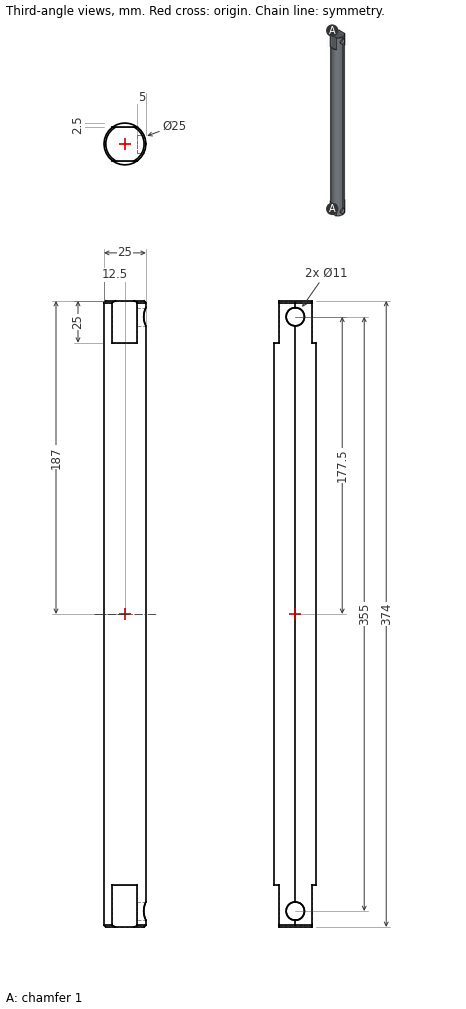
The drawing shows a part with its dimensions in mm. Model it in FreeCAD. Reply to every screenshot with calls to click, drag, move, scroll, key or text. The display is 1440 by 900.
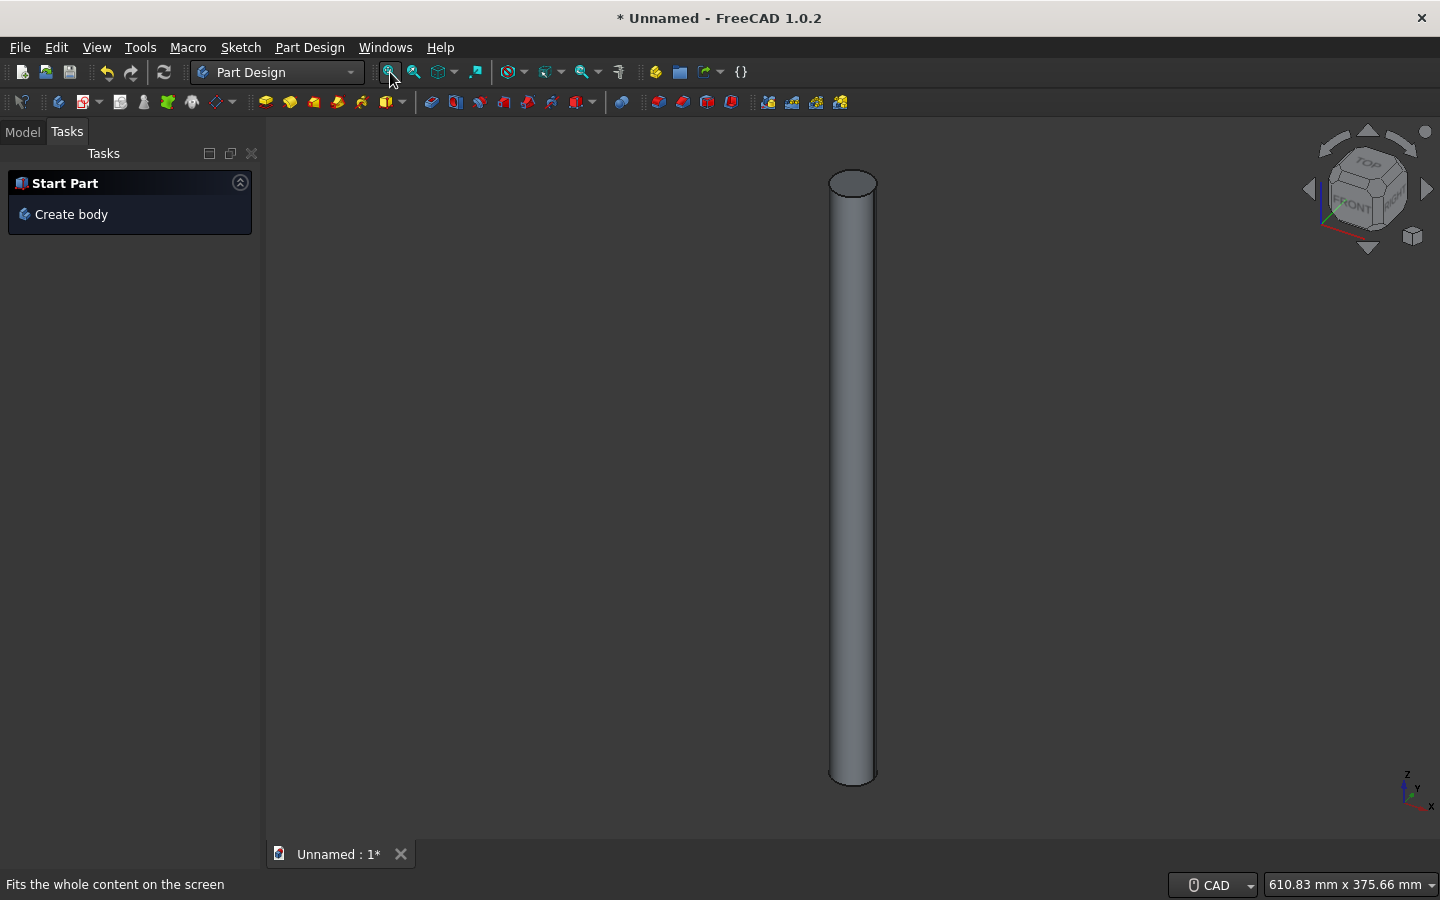
click(835, 781)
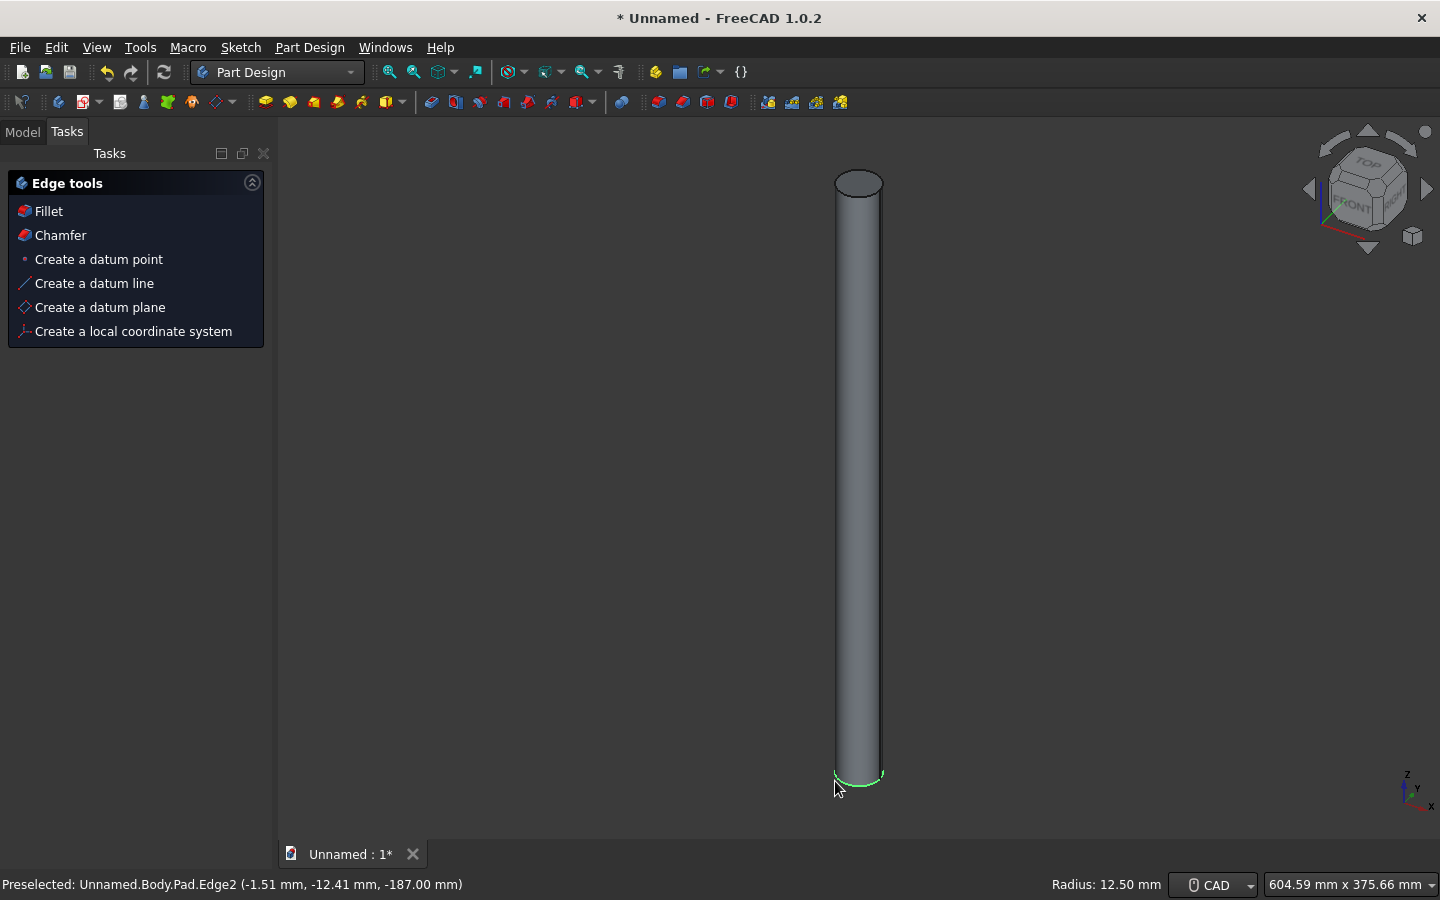
click(835, 184, ctrl)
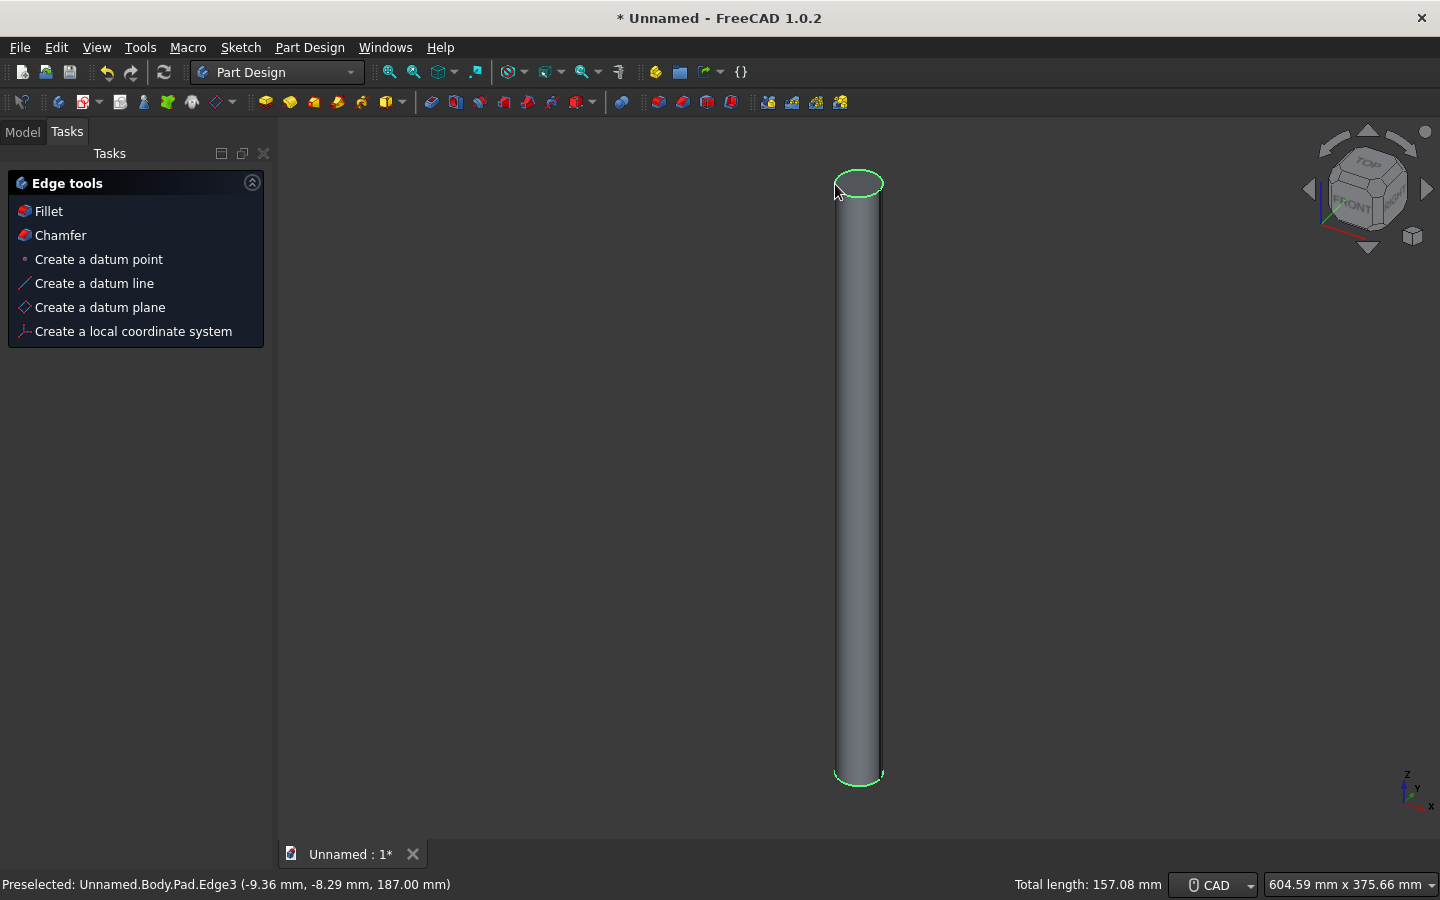
click(684, 102)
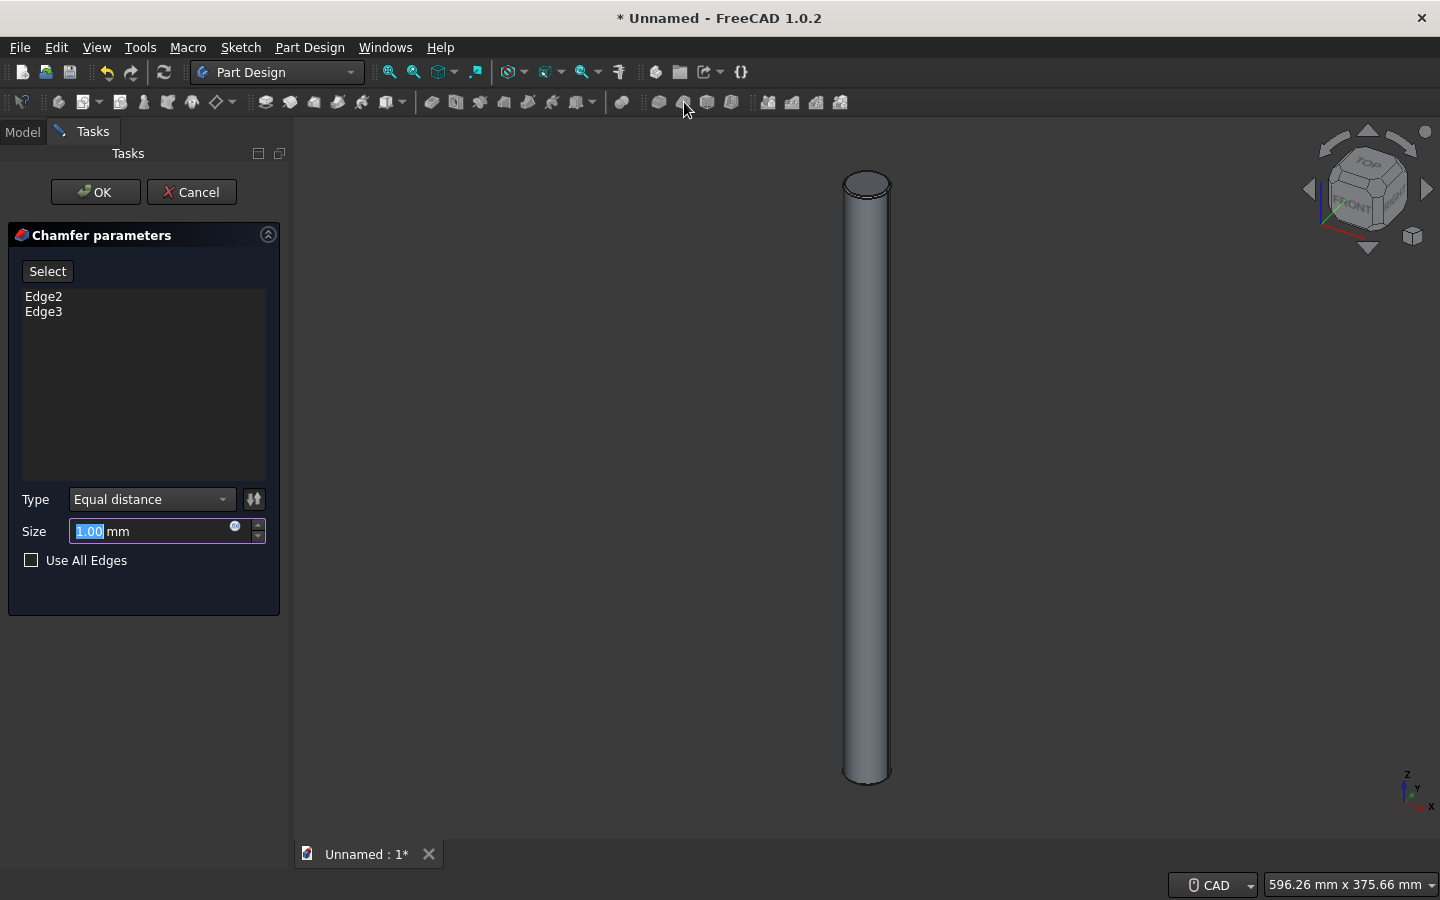
text(1)
key(Tab)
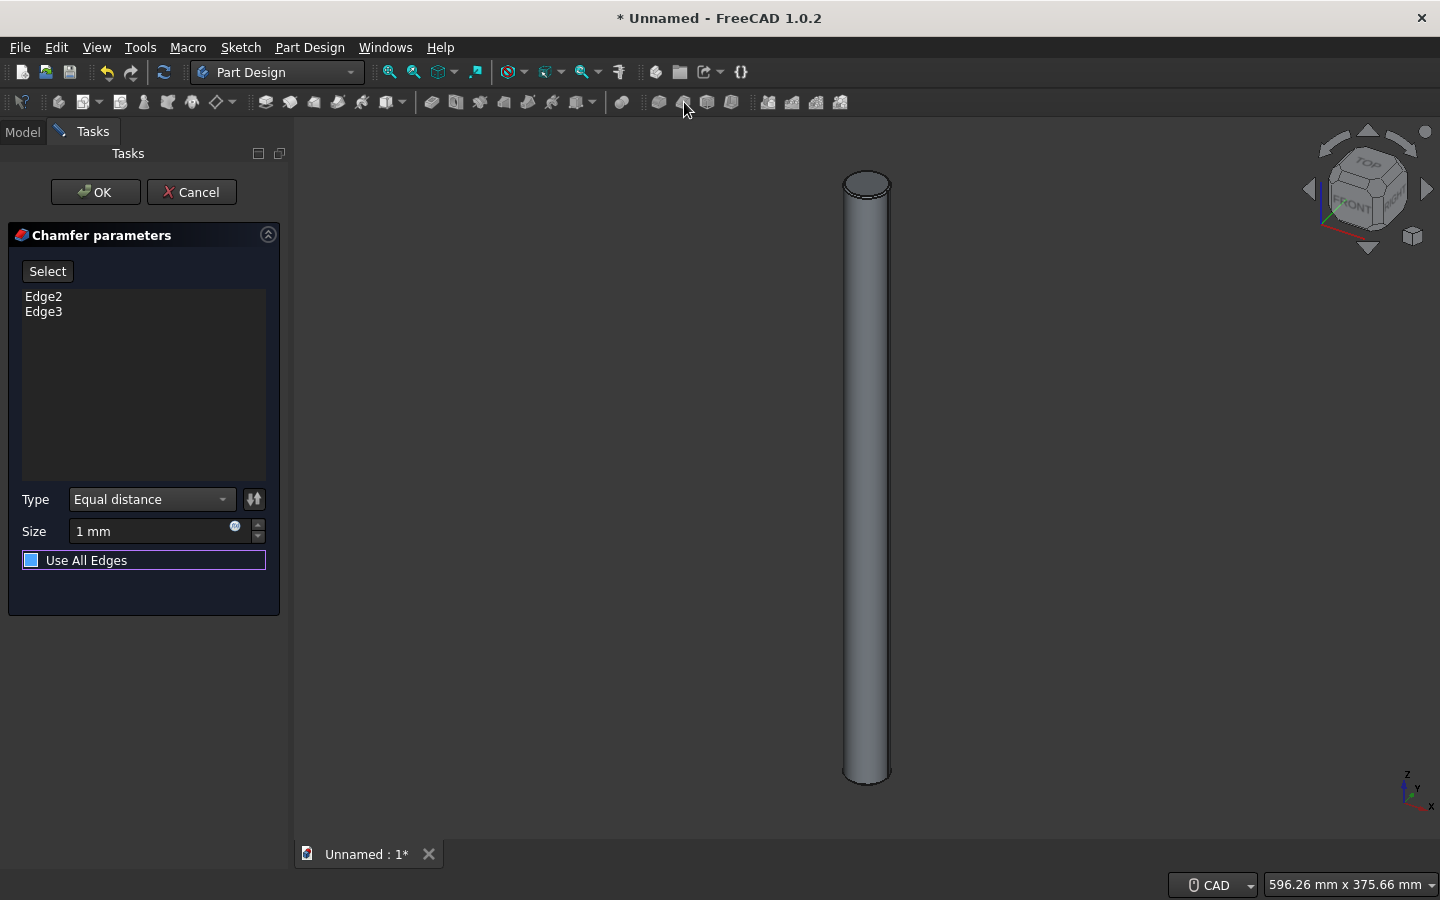
click(96, 192)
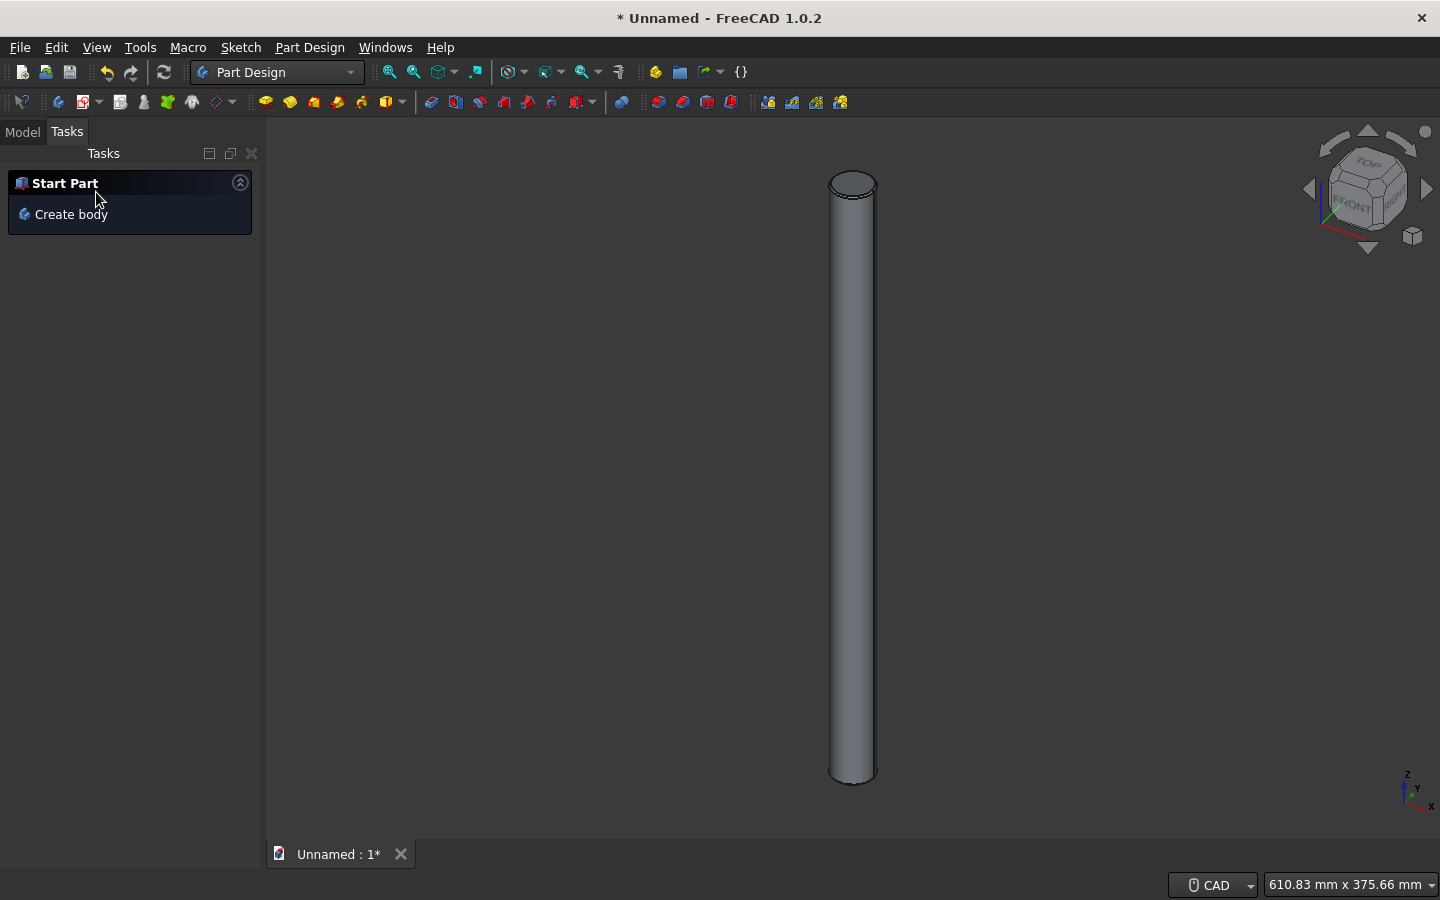
click(23, 131)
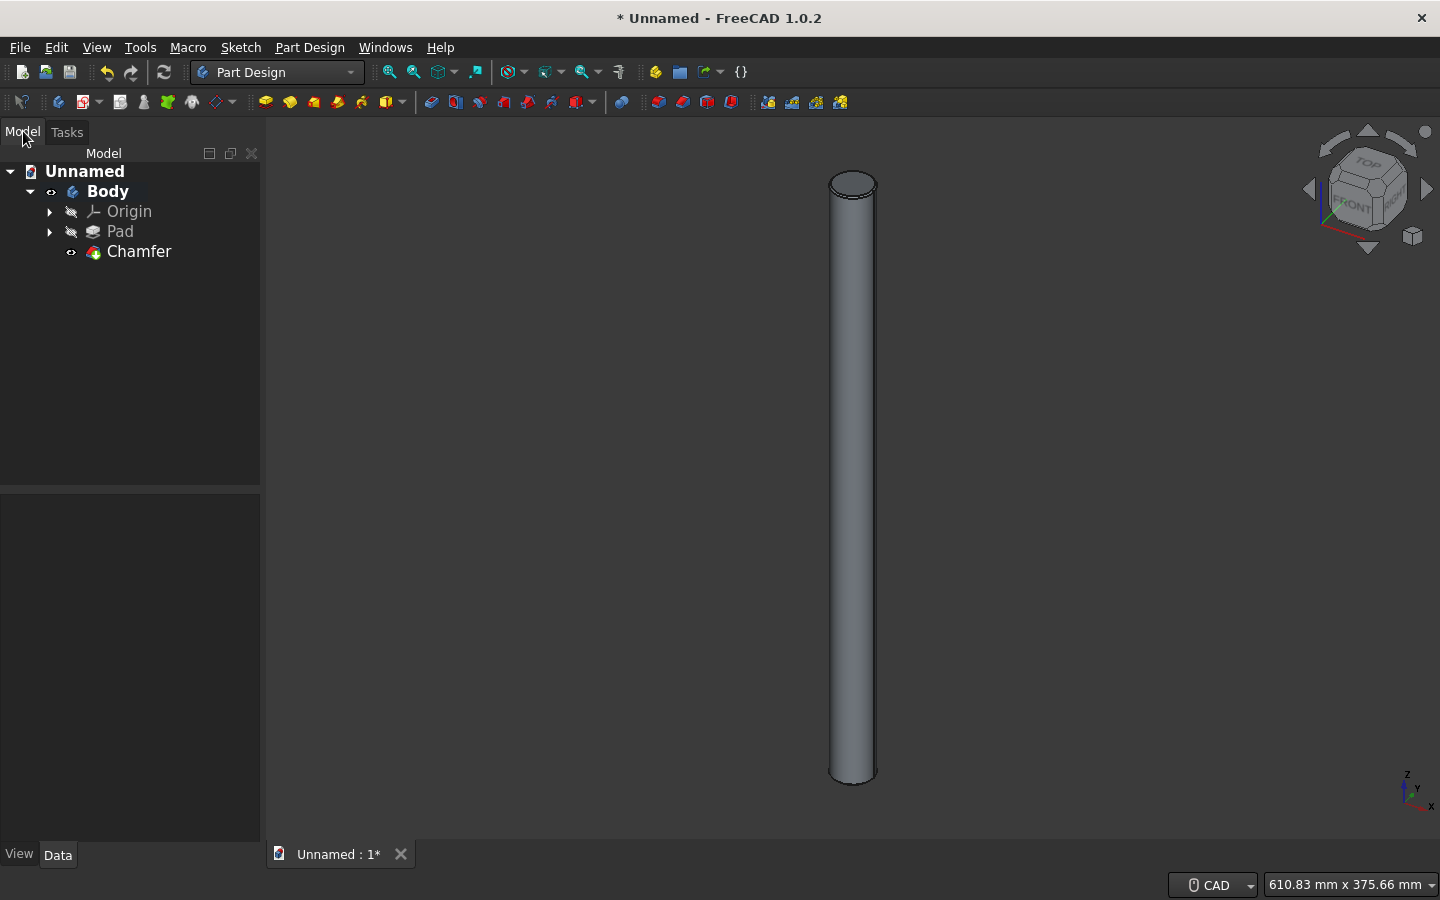
click(50, 212)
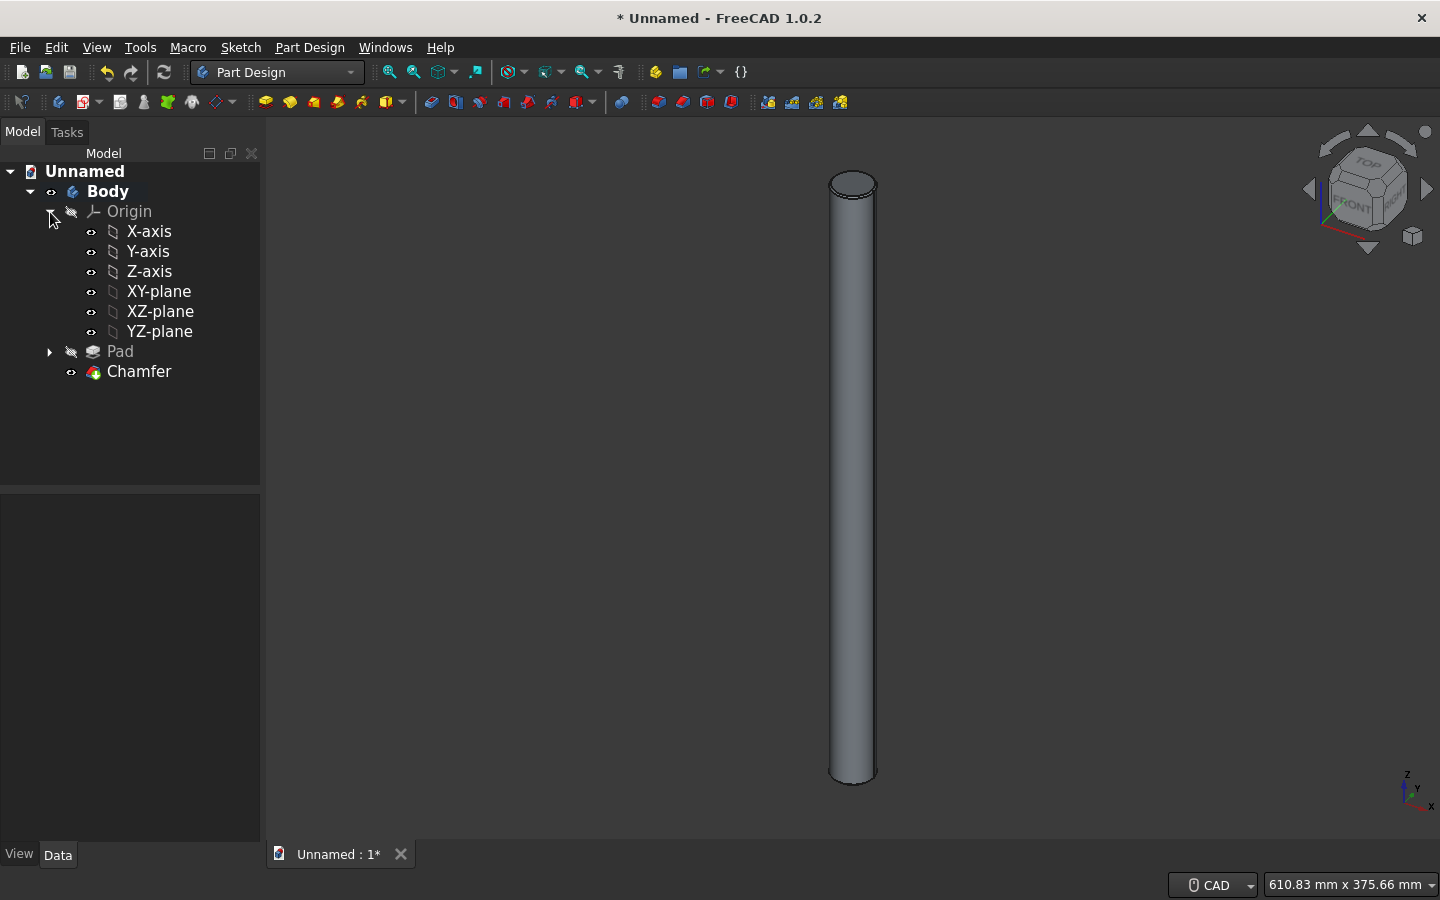
click(136, 312)